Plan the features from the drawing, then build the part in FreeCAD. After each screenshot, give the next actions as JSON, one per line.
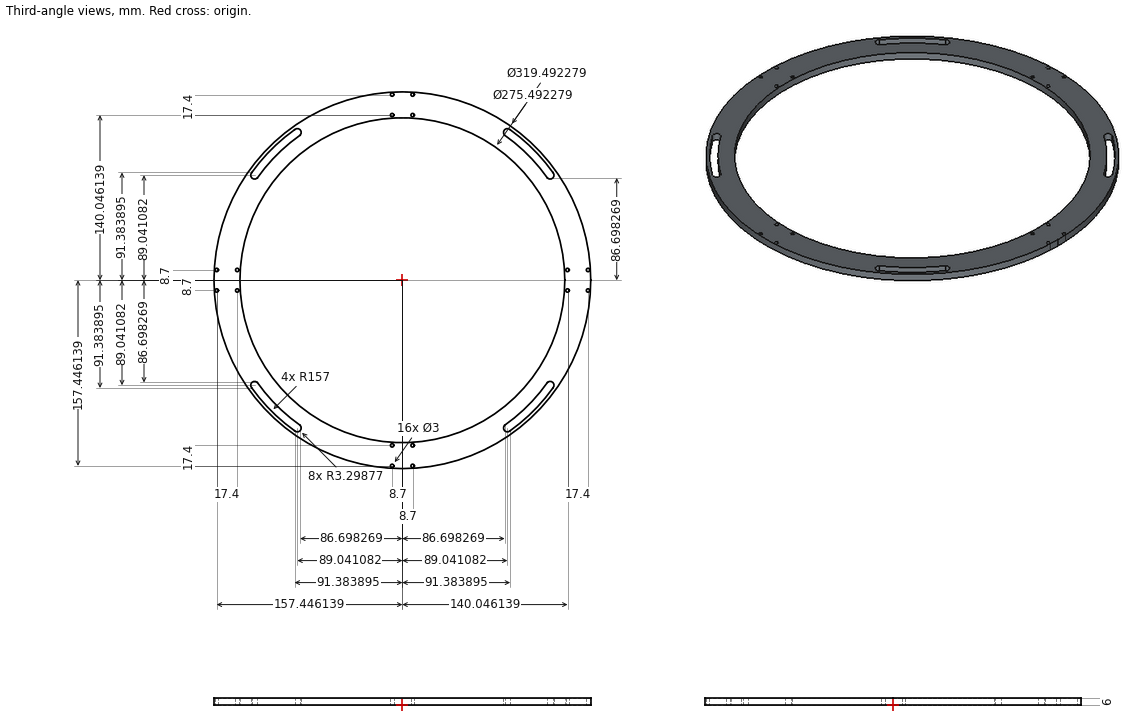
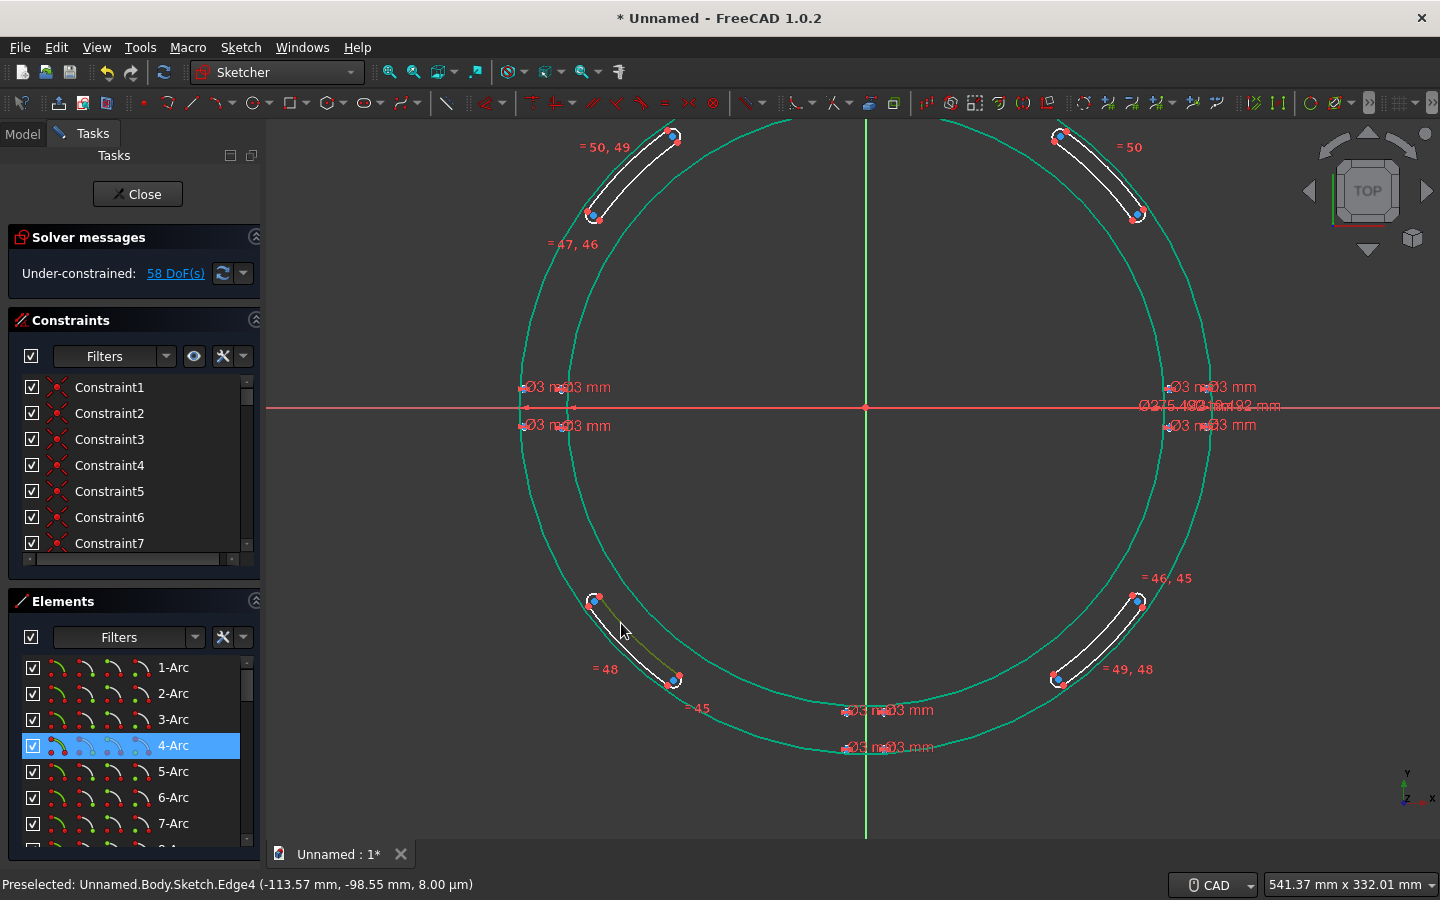
{"action": "left_click", "coordinate": [1080, 653]}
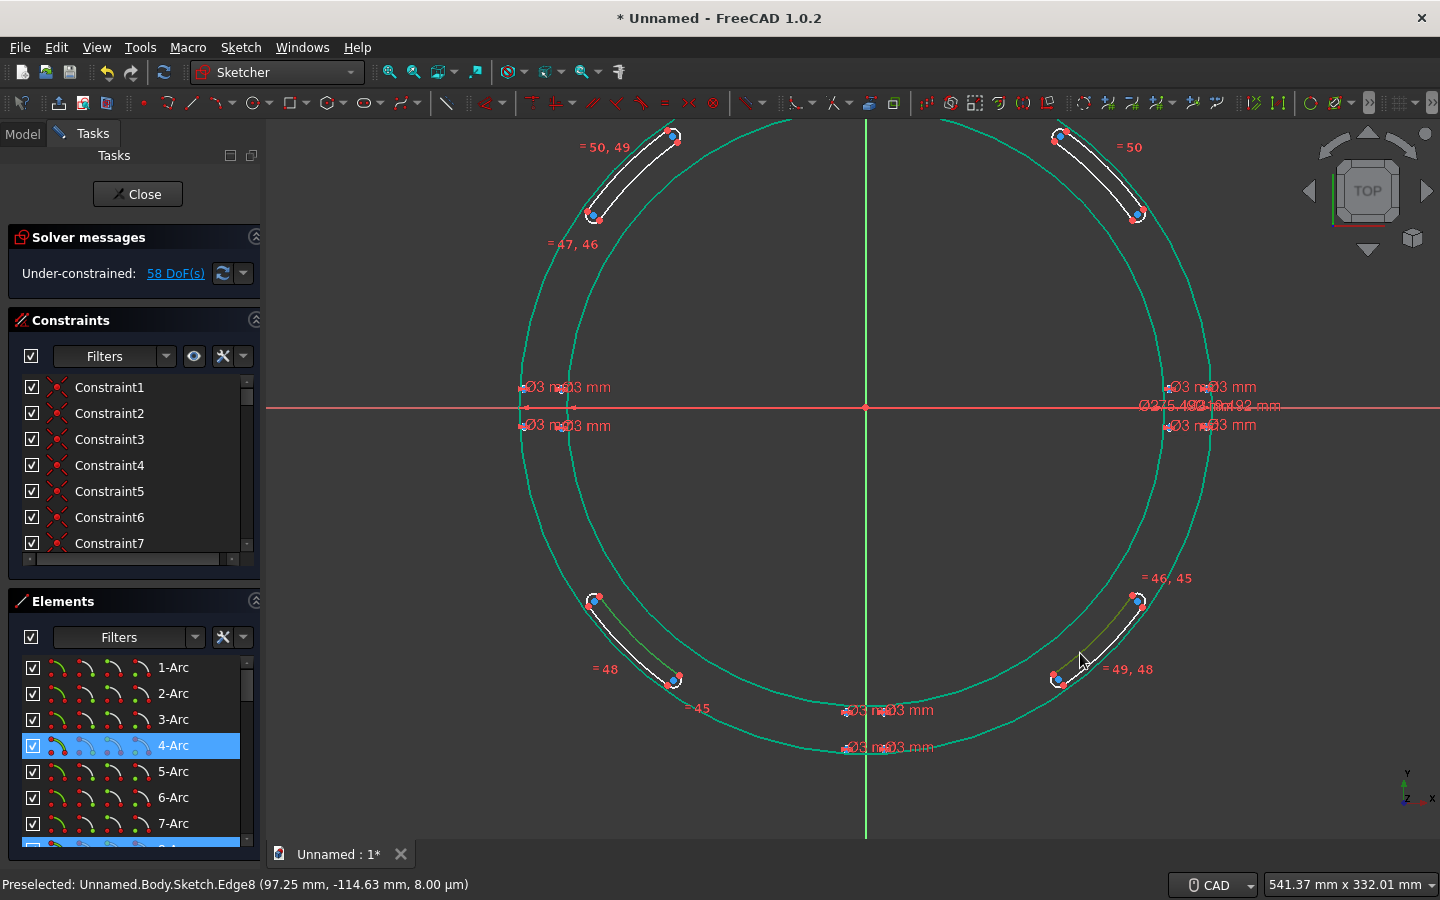
{"action": "left_click", "coordinate": [652, 163]}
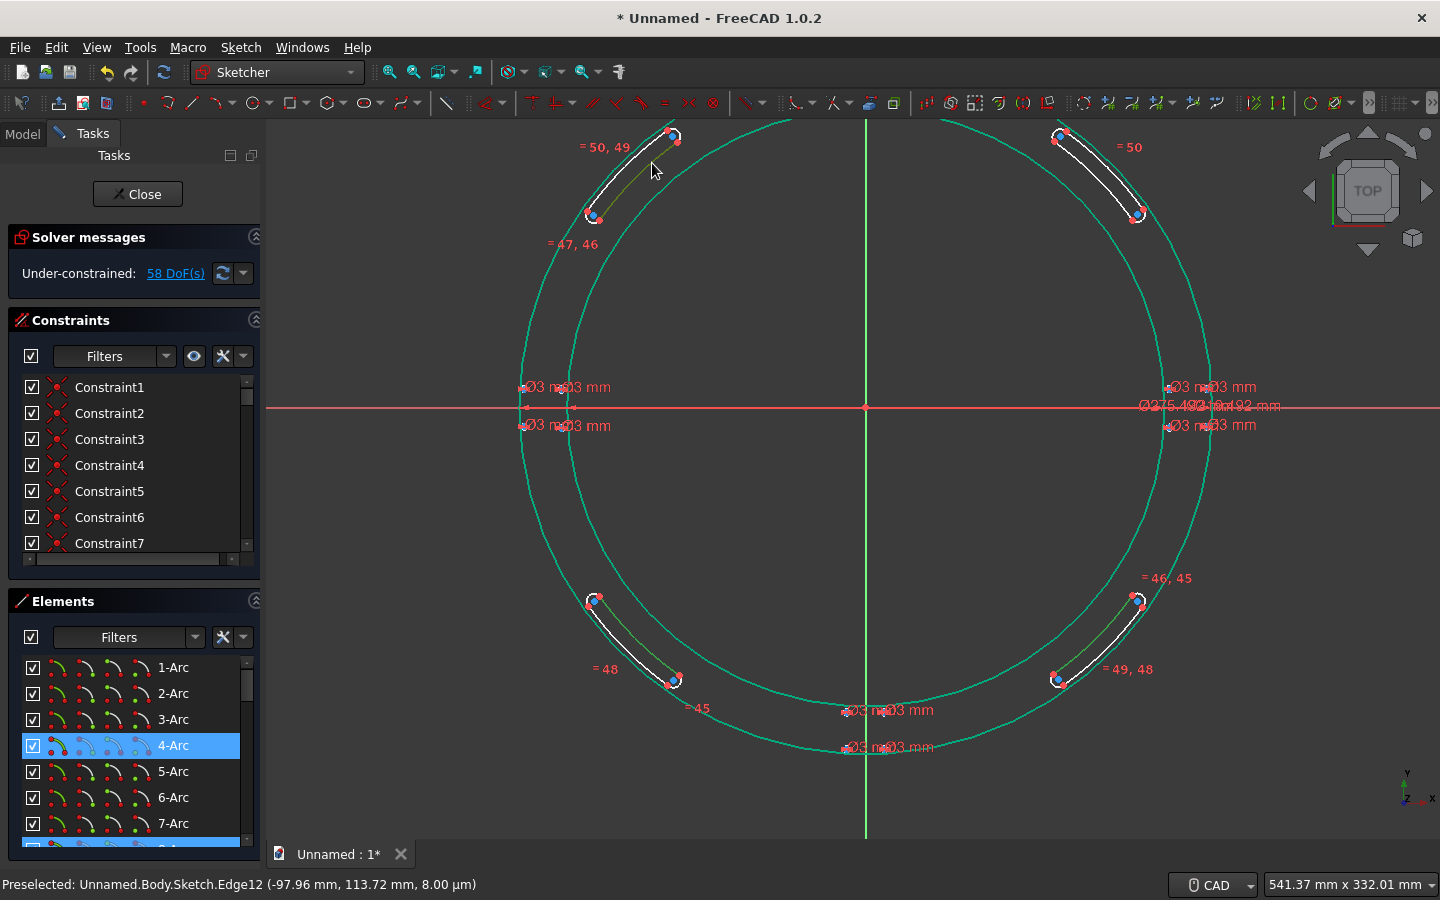
{"action": "left_click", "coordinate": [1112, 194]}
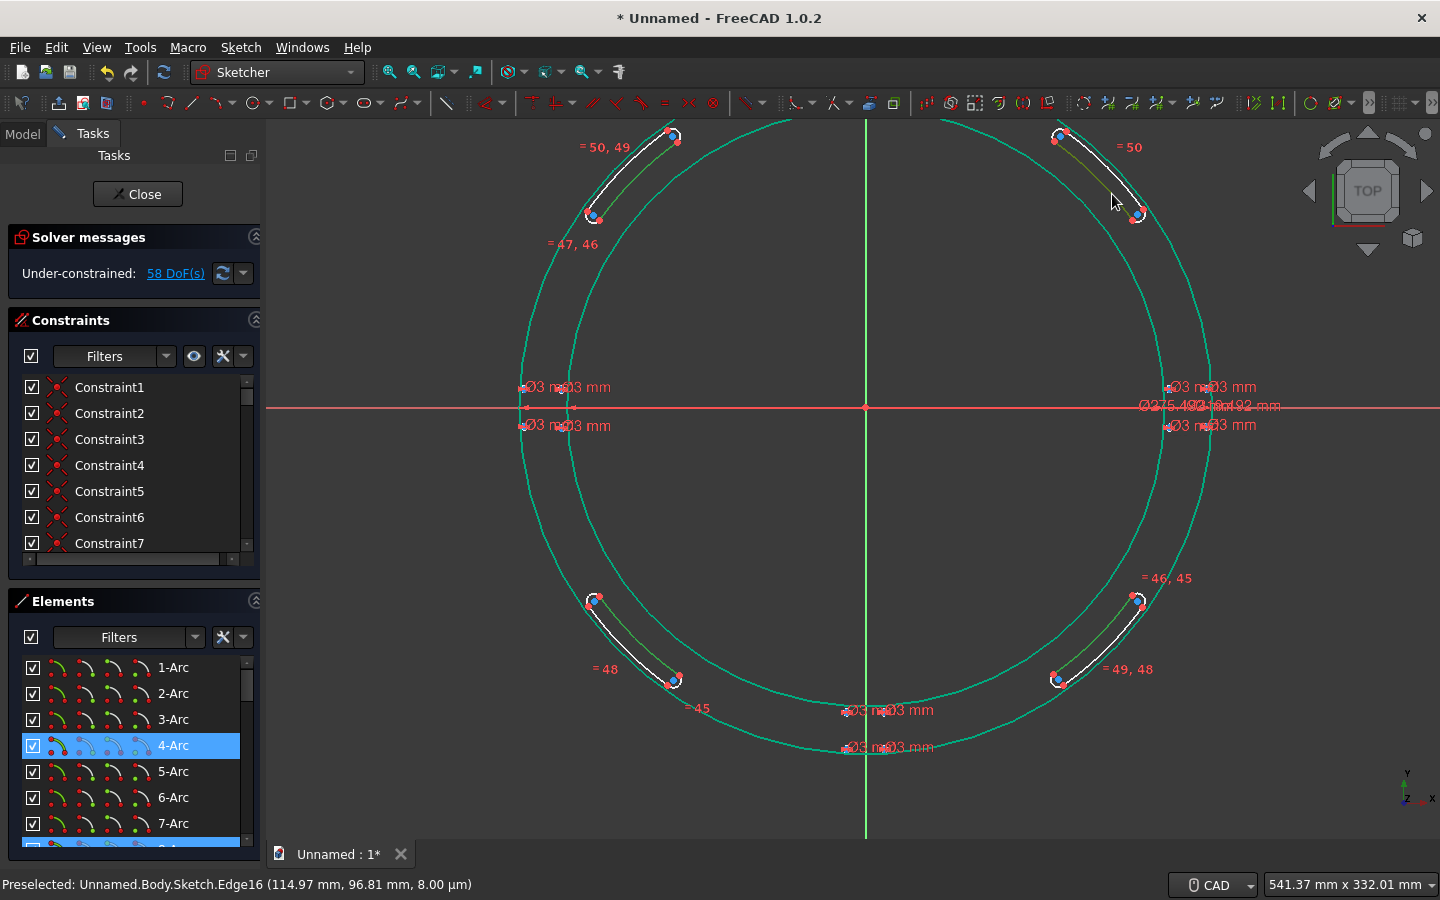
{"action": "key", "text": "e"}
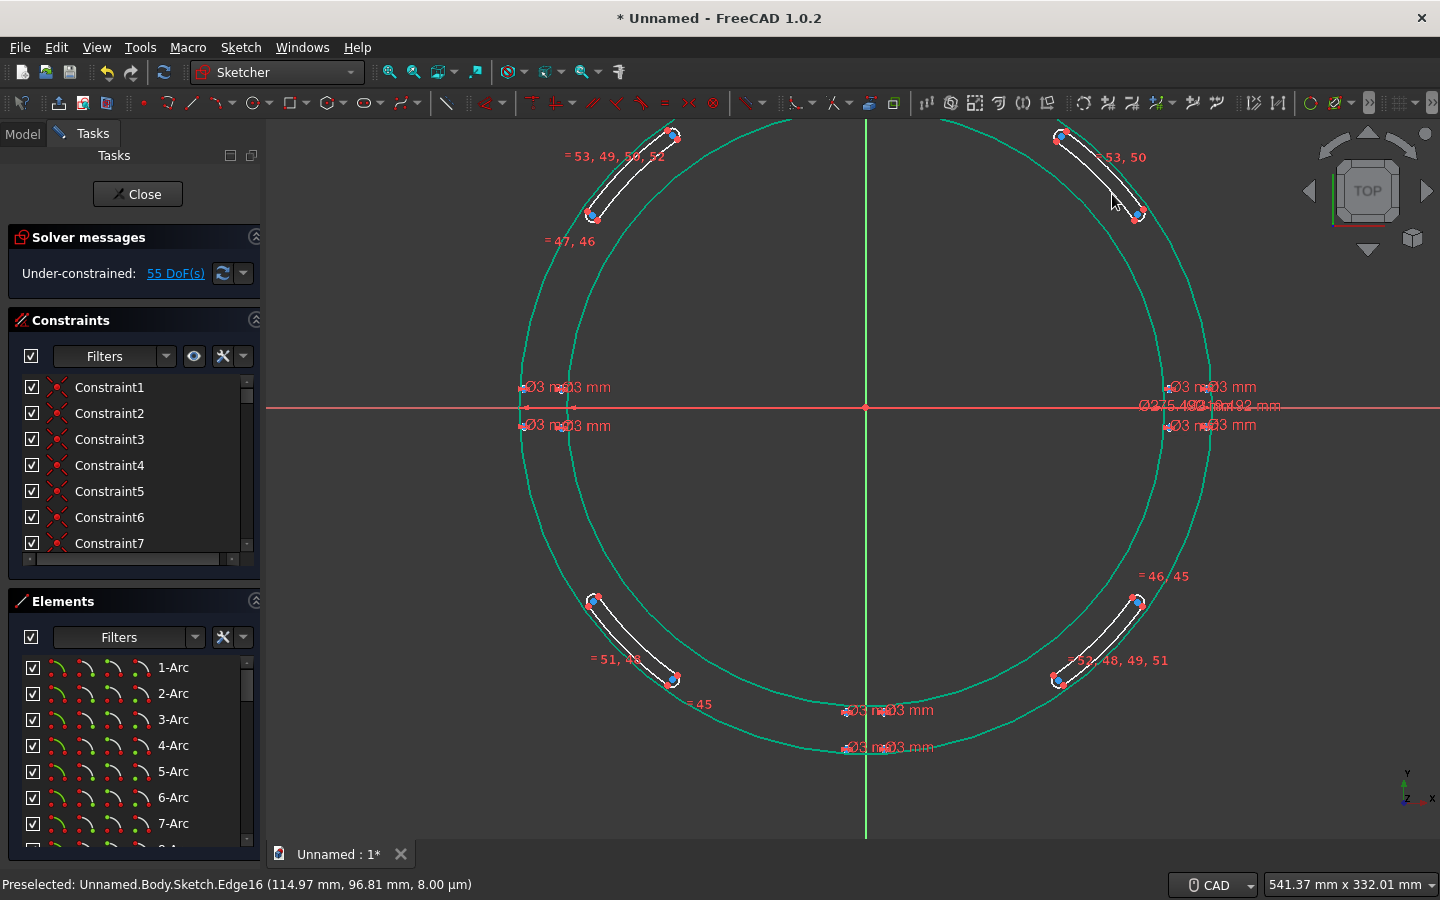
{"action": "left_click", "coordinate": [847, 749]}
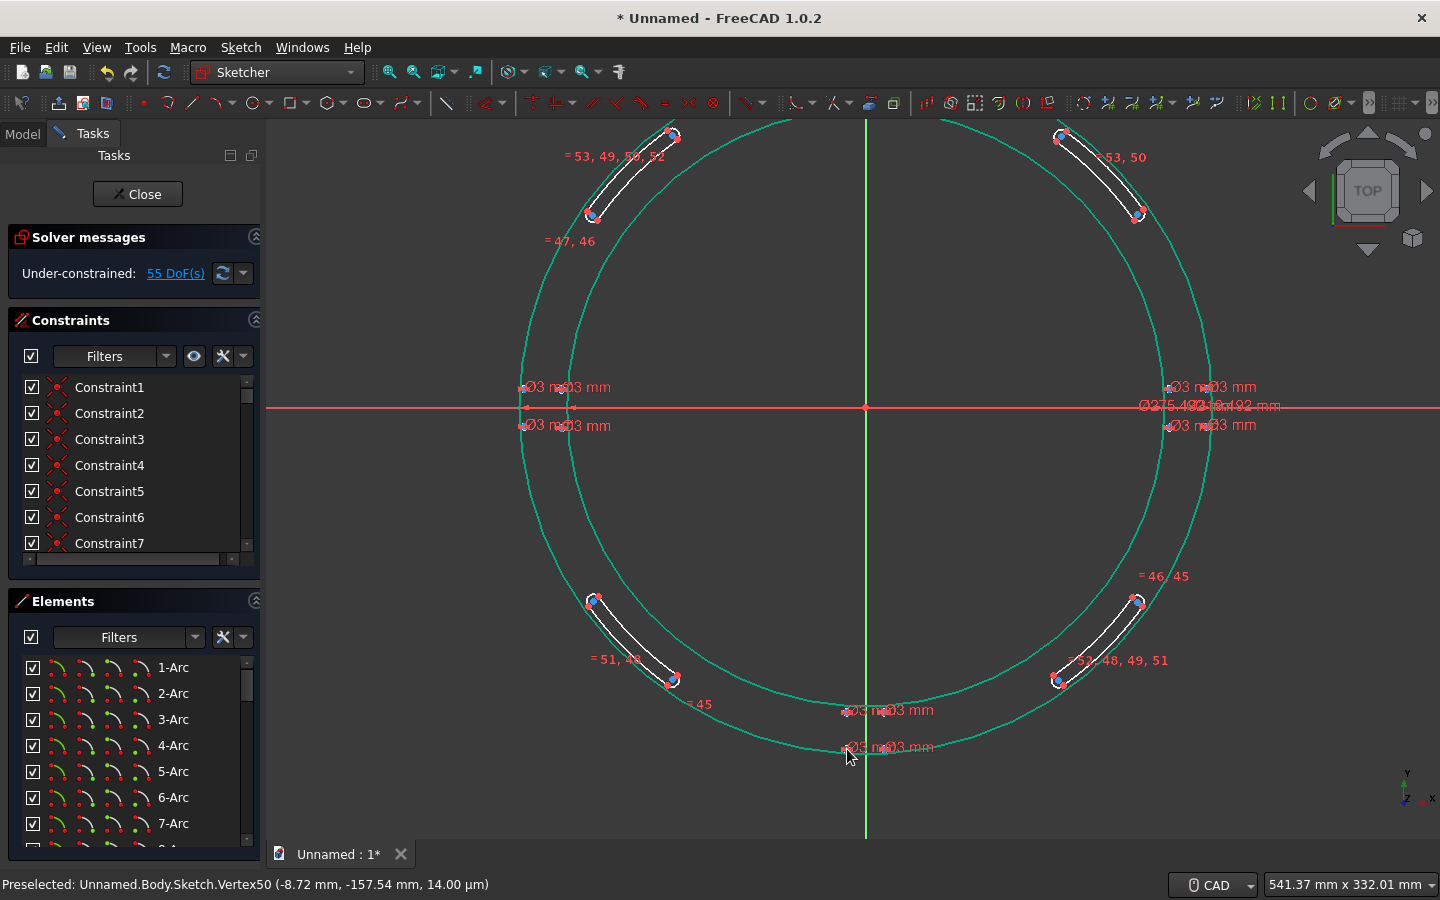
{"action": "left_click", "coordinate": [847, 712]}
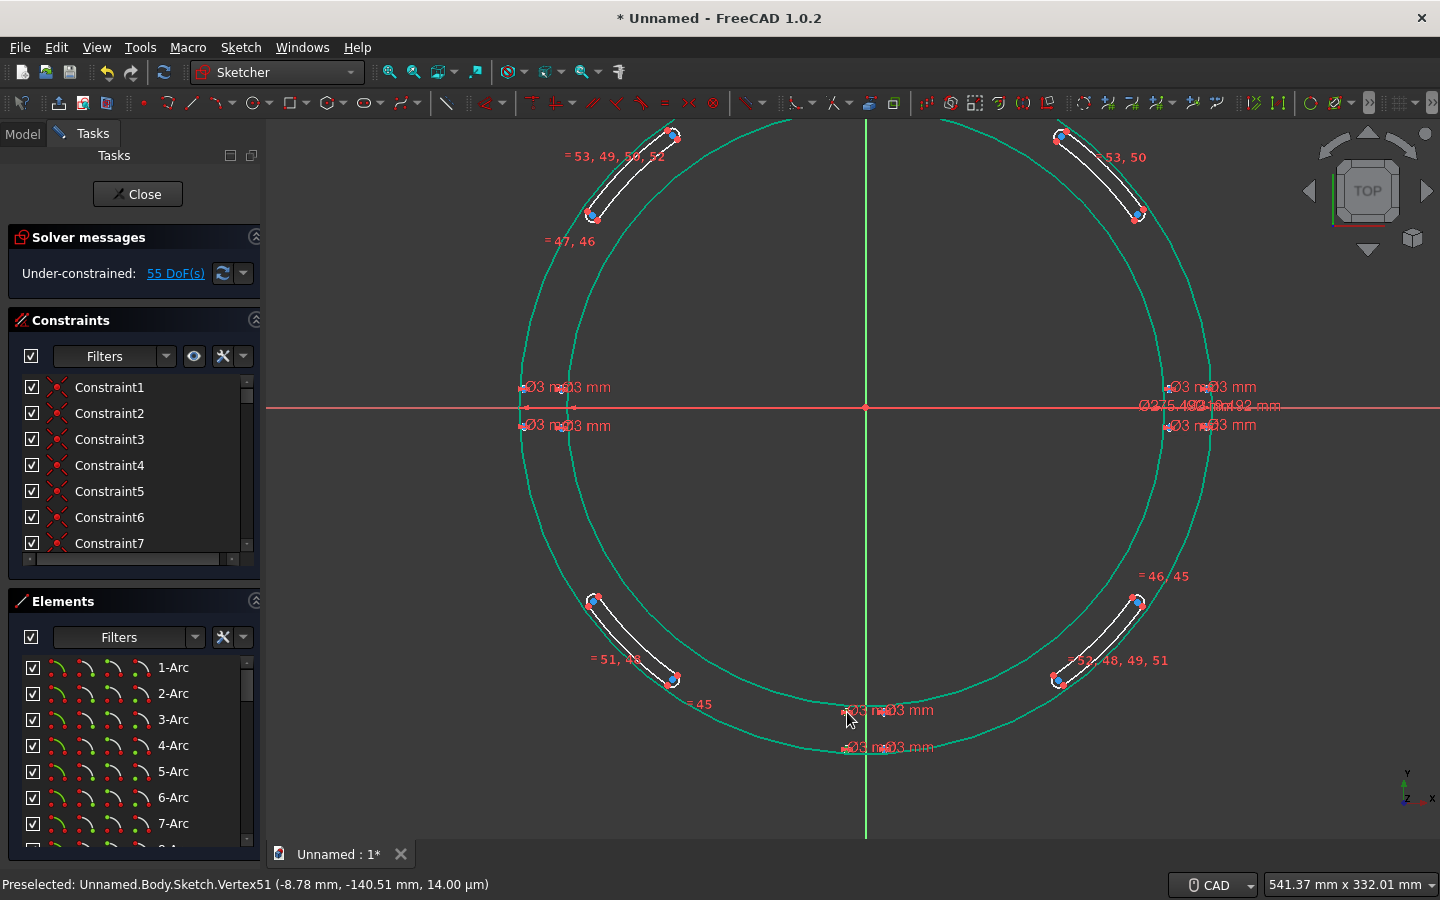
{"action": "left_click", "coordinate": [574, 104]}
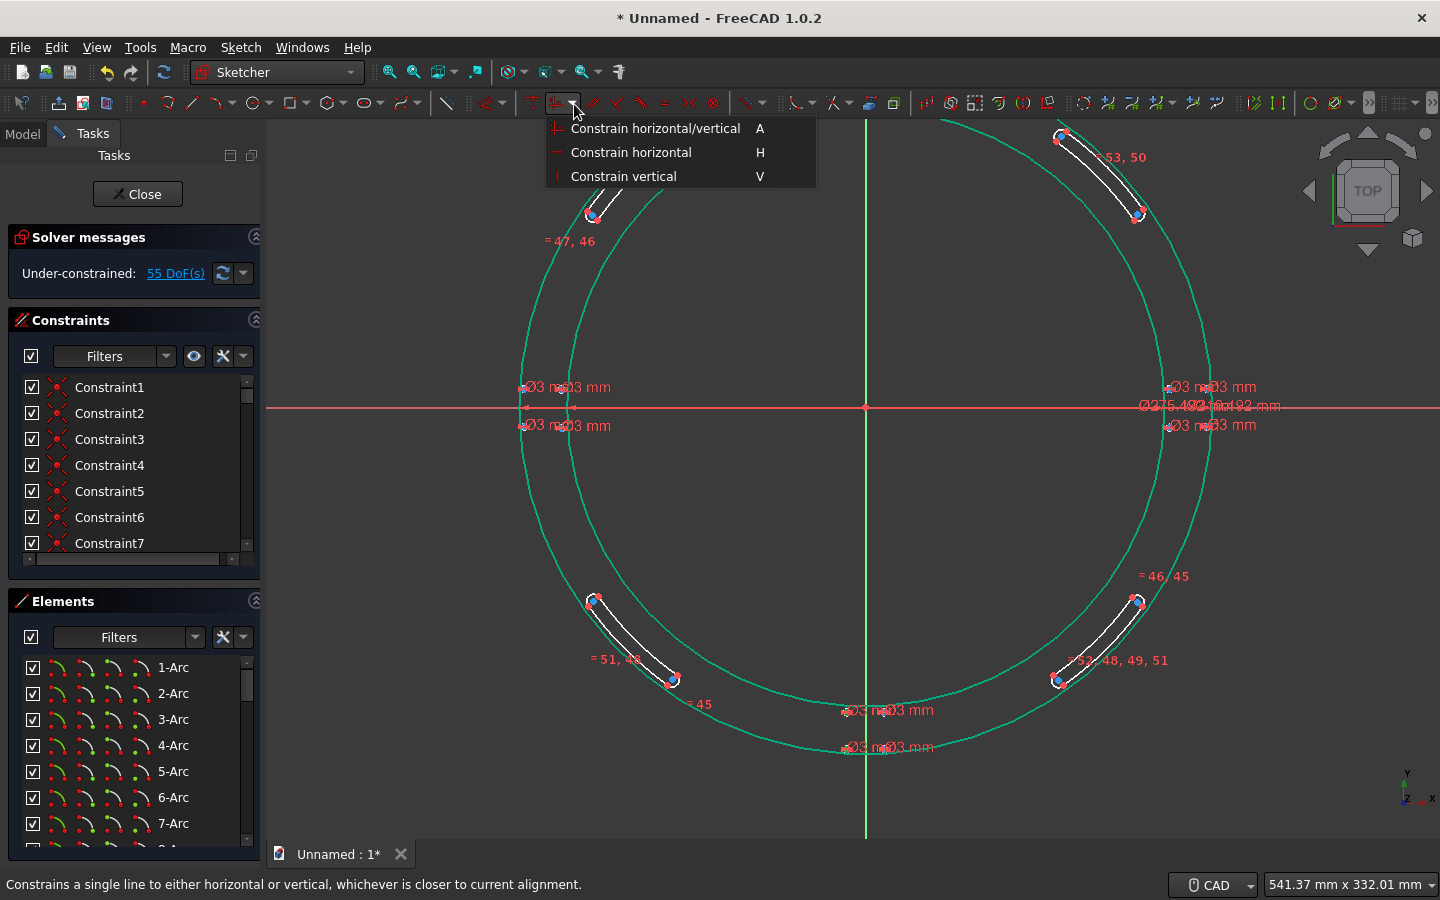
{"action": "left_click", "coordinate": [681, 176]}